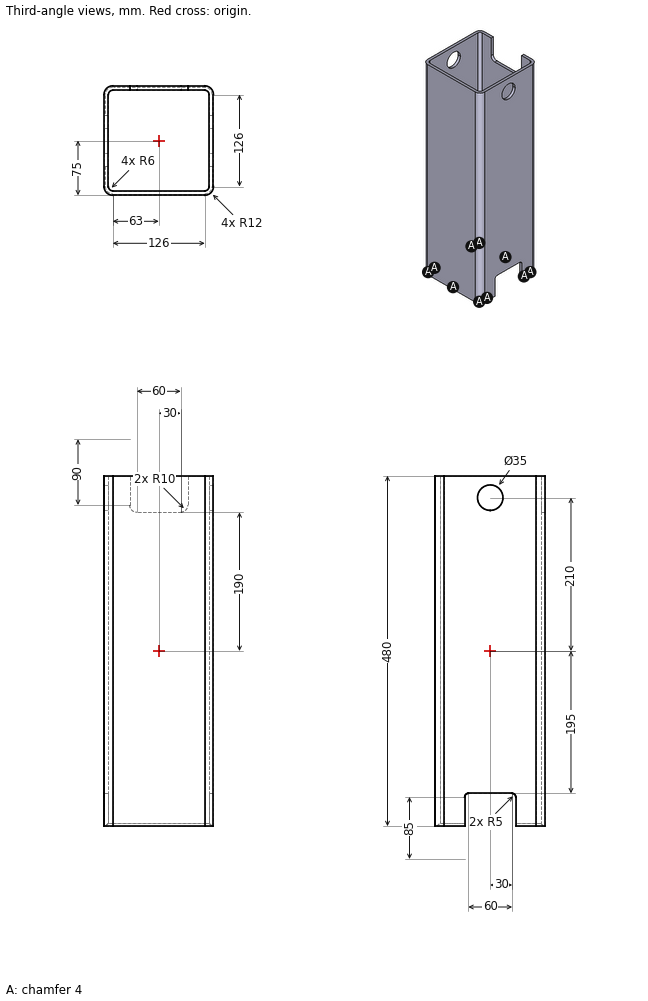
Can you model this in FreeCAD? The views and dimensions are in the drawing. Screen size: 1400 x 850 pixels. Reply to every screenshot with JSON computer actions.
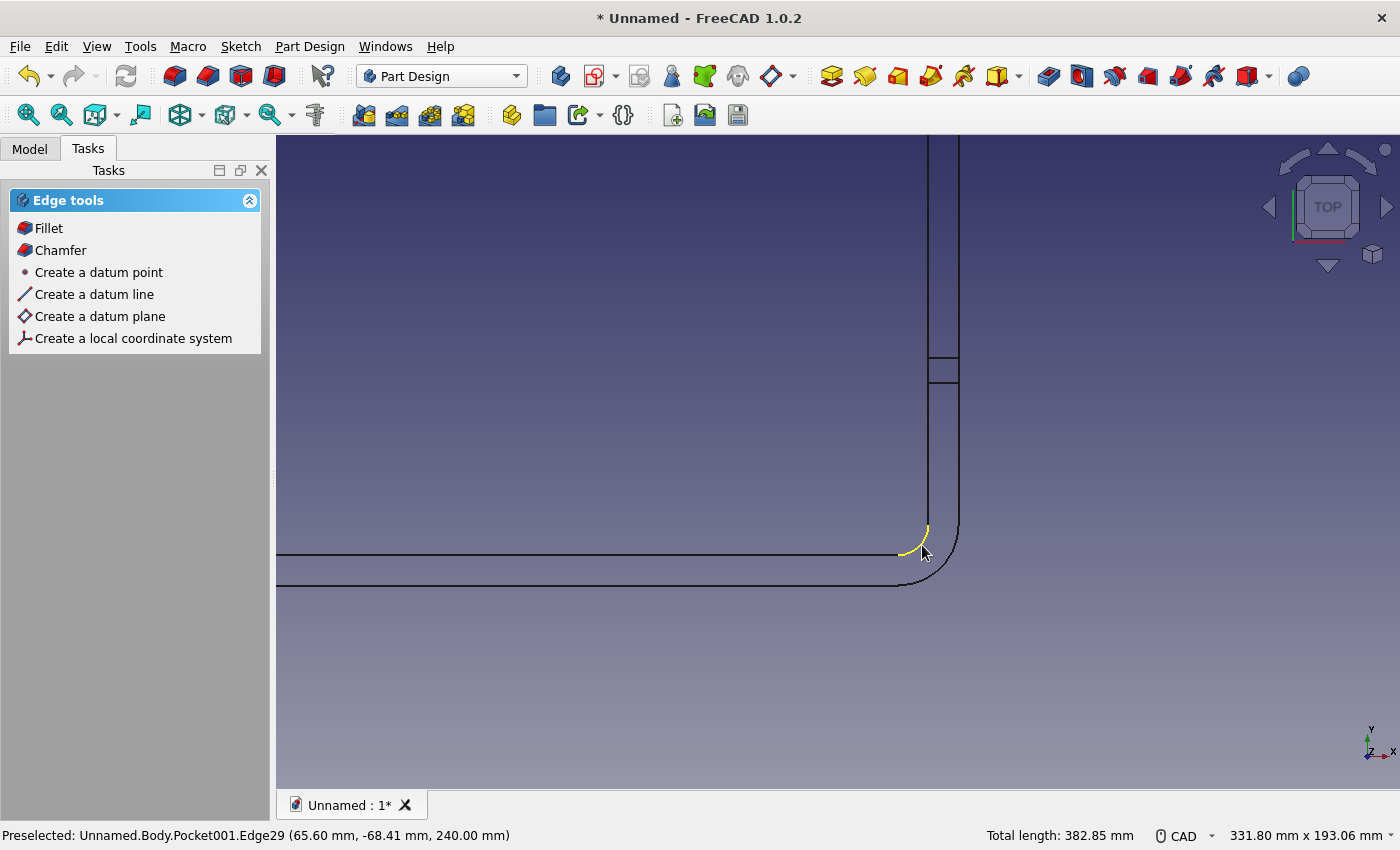
{"action": "key", "text": "v f"}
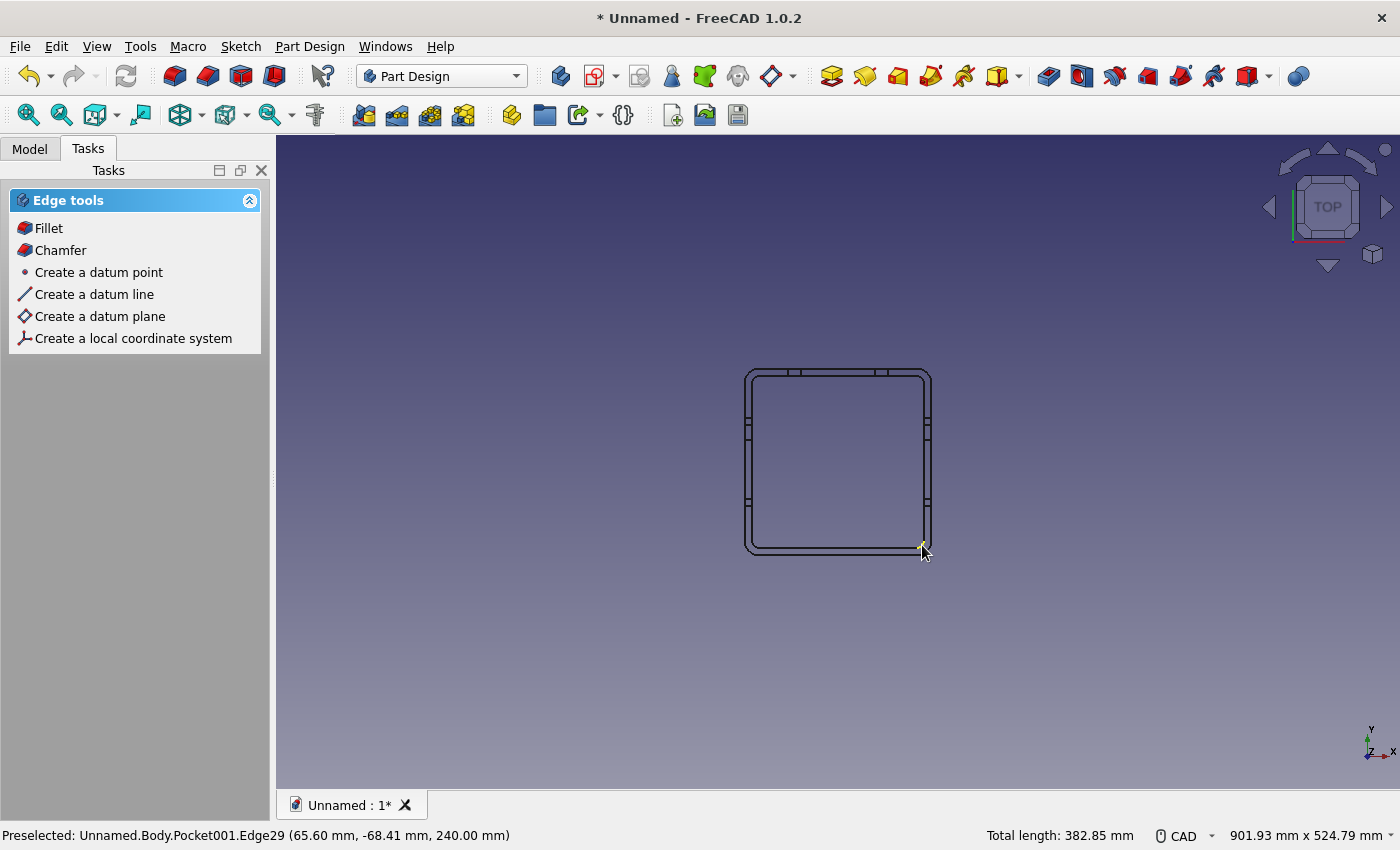
{"action": "key", "text": "1"}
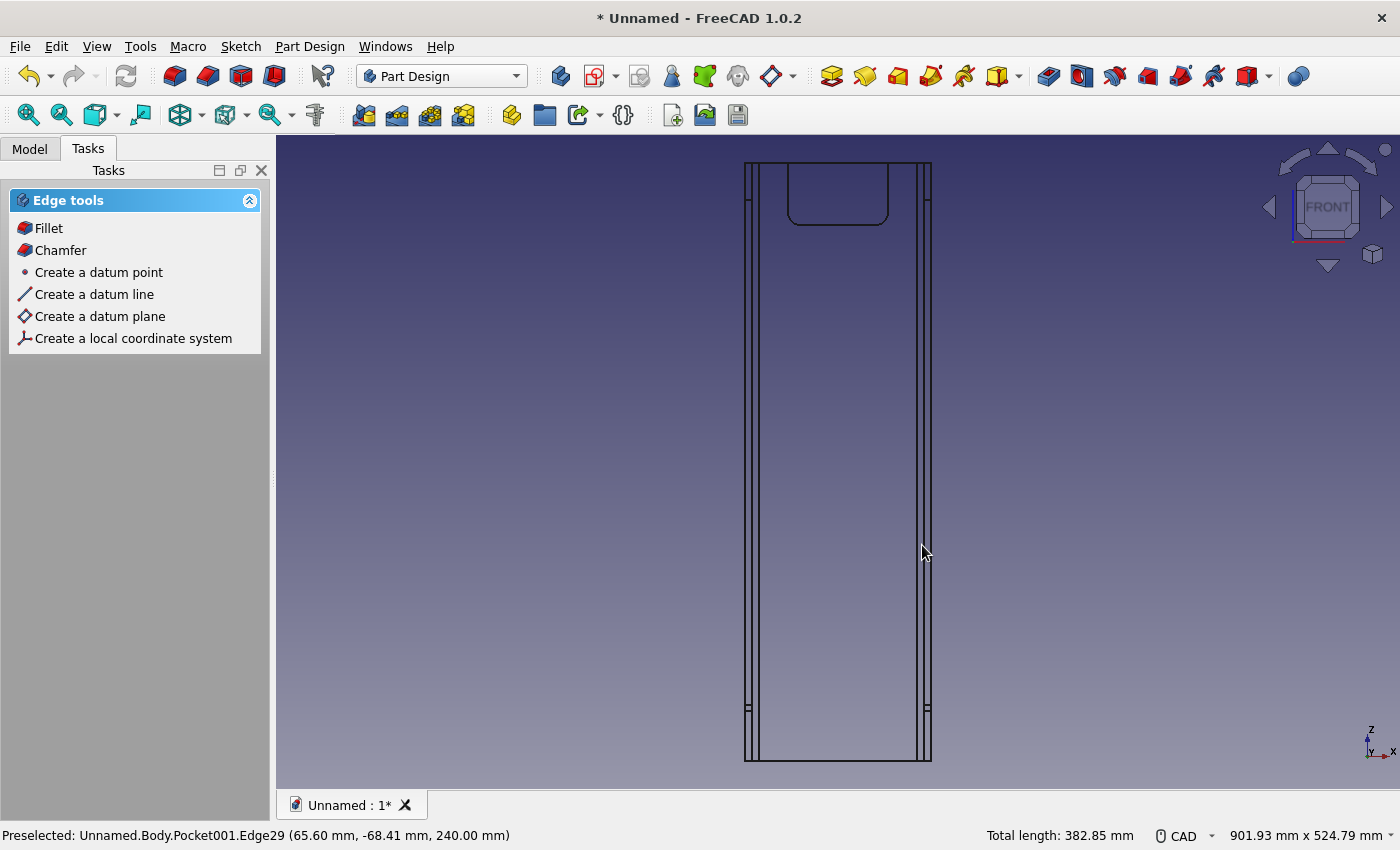
{"action": "scroll", "coordinate": [922, 760], "scroll_direction": "up", "scroll_amount": 7}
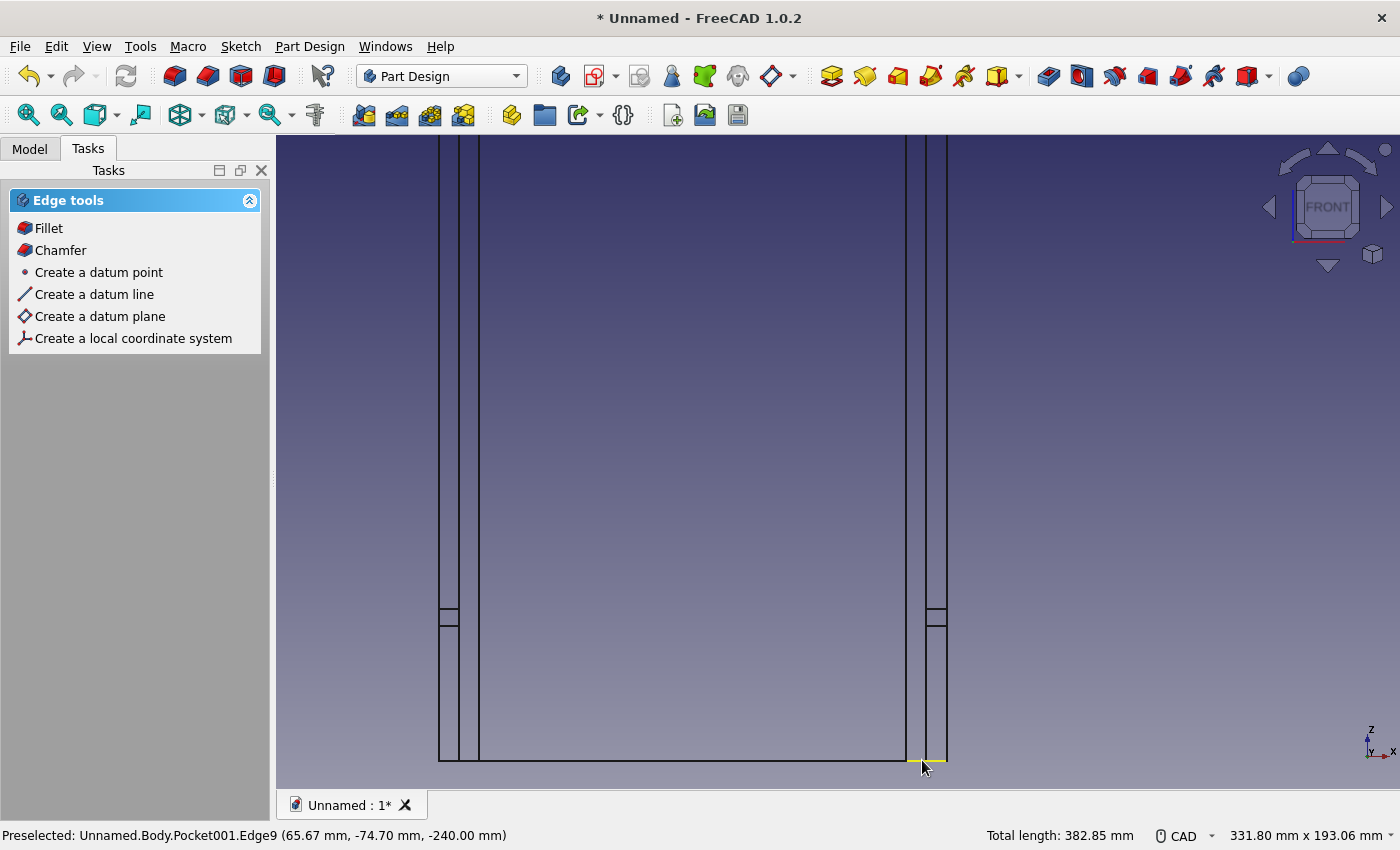
{"action": "key", "text": "v f"}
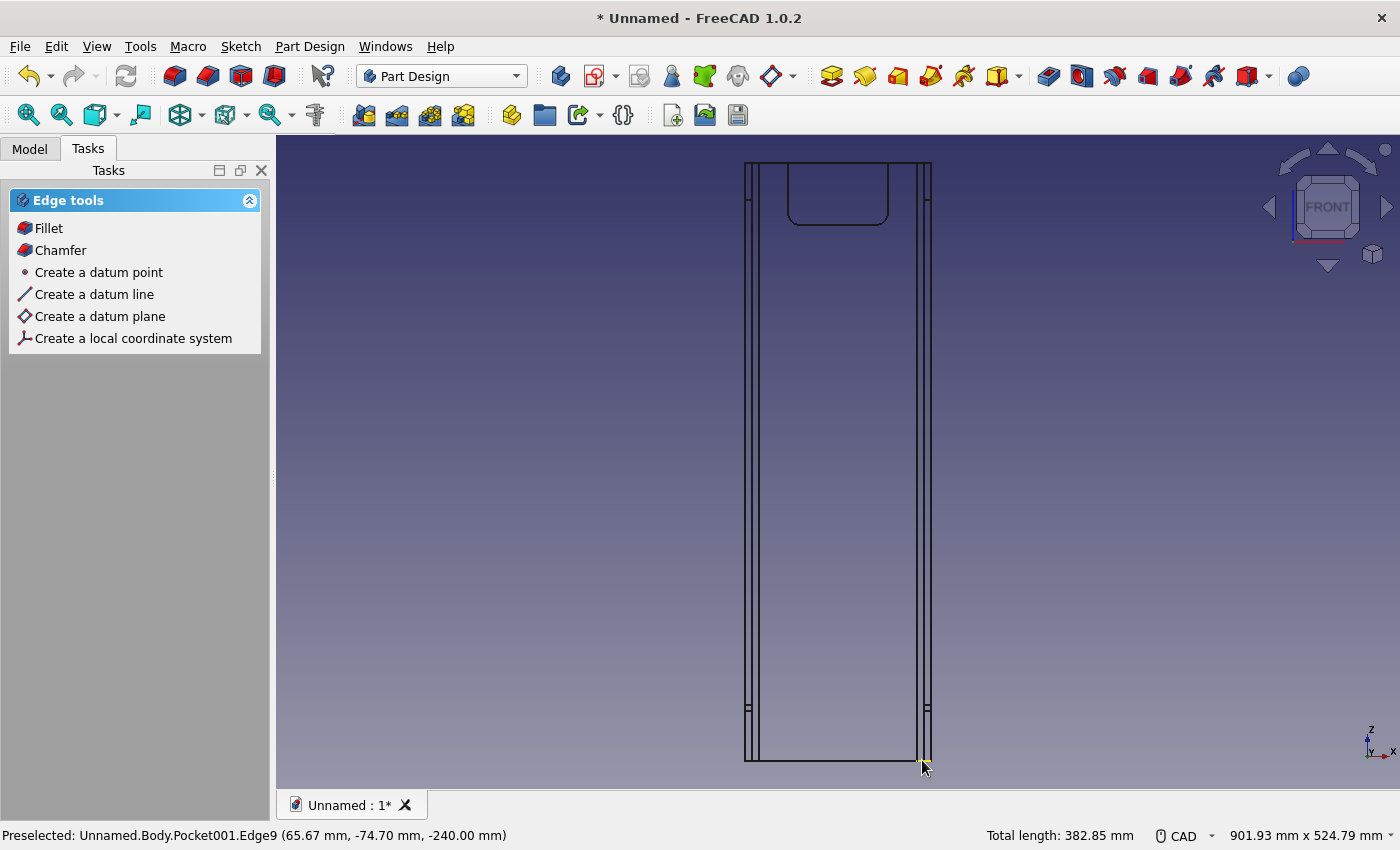
{"action": "key", "text": "3"}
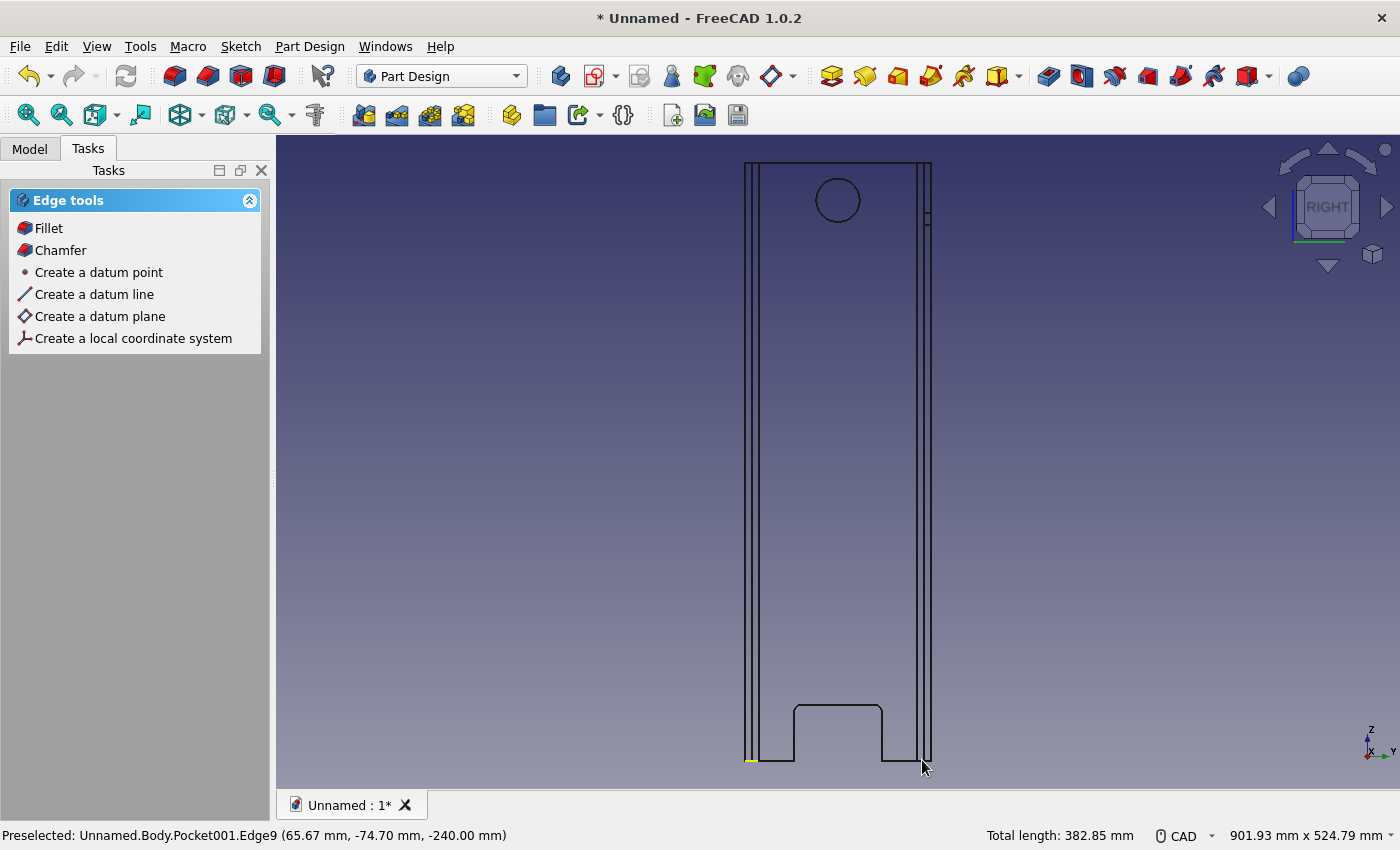
{"action": "scroll", "coordinate": [754, 760], "scroll_direction": "up", "scroll_amount": 7}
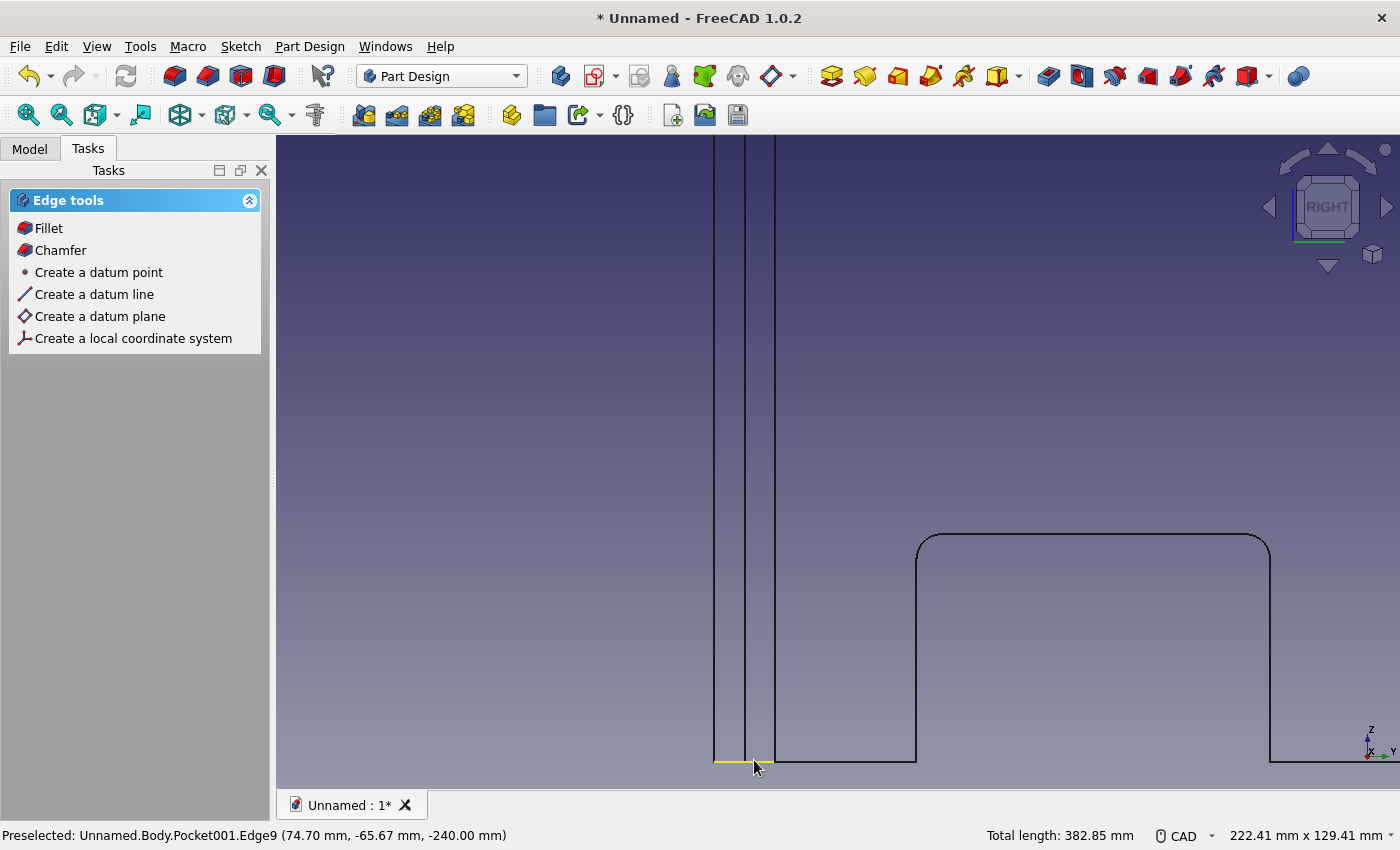
{"action": "left_click", "coordinate": [29, 116]}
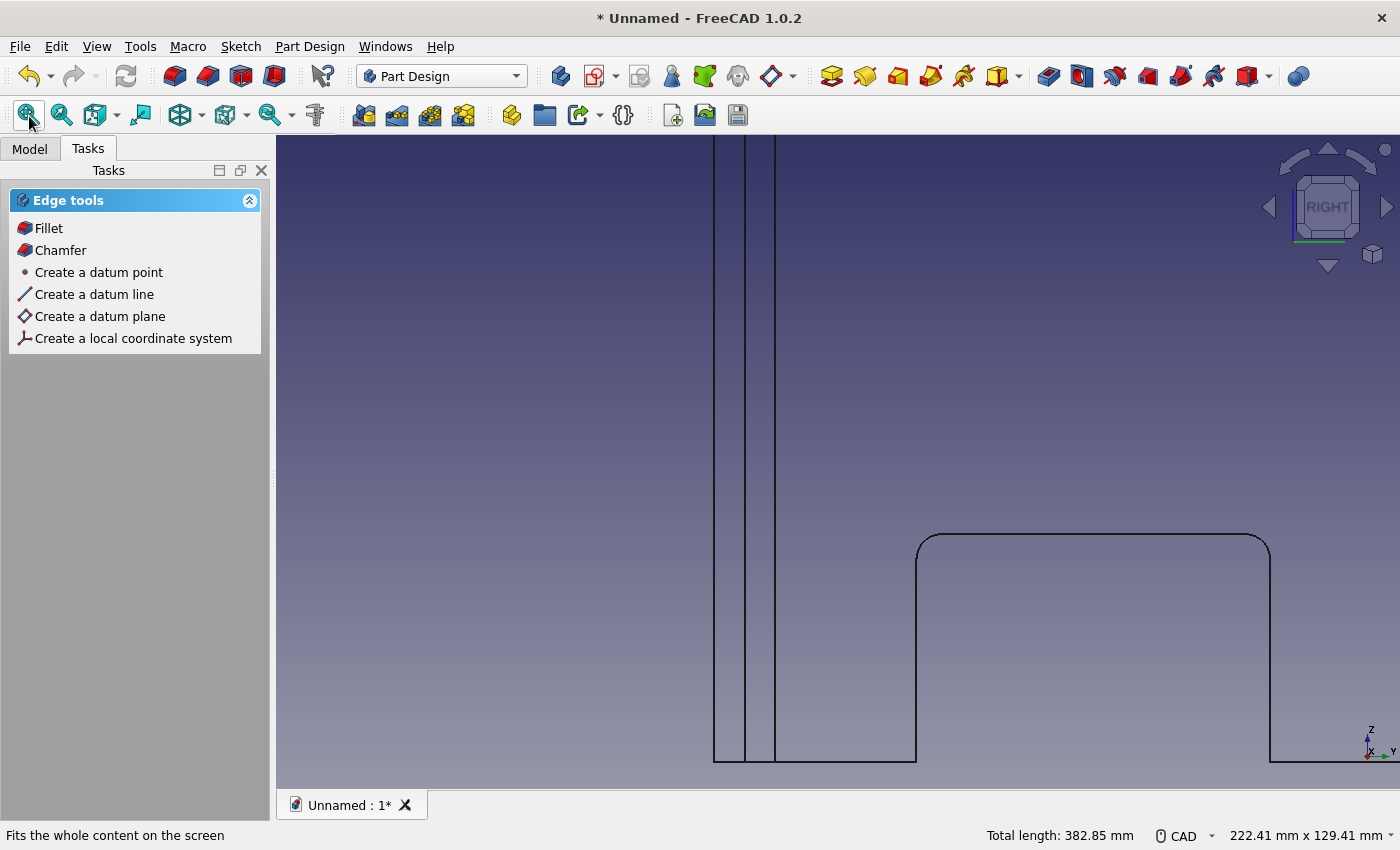
{"action": "key", "text": "5"}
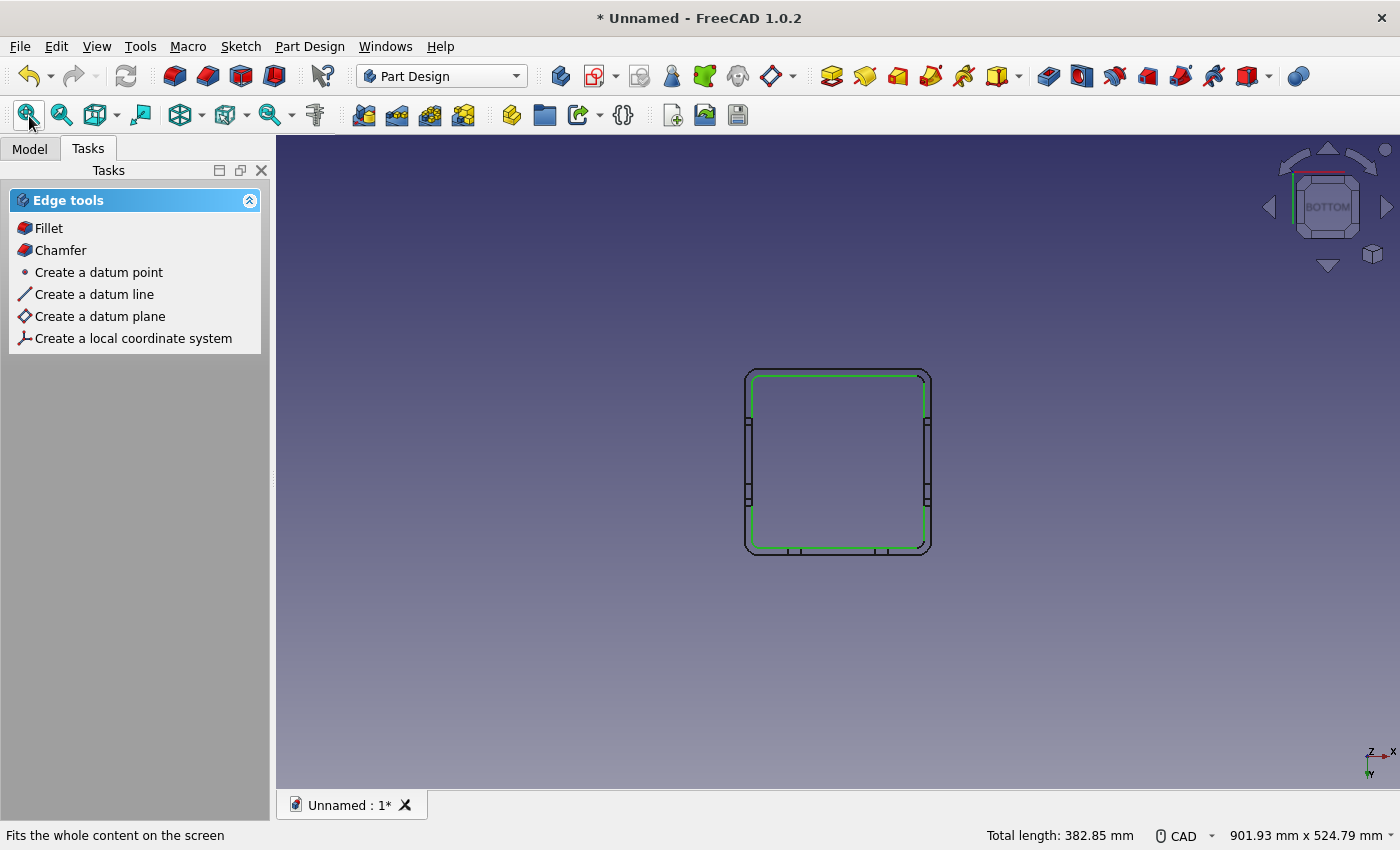
{"action": "key", "text": "v f"}